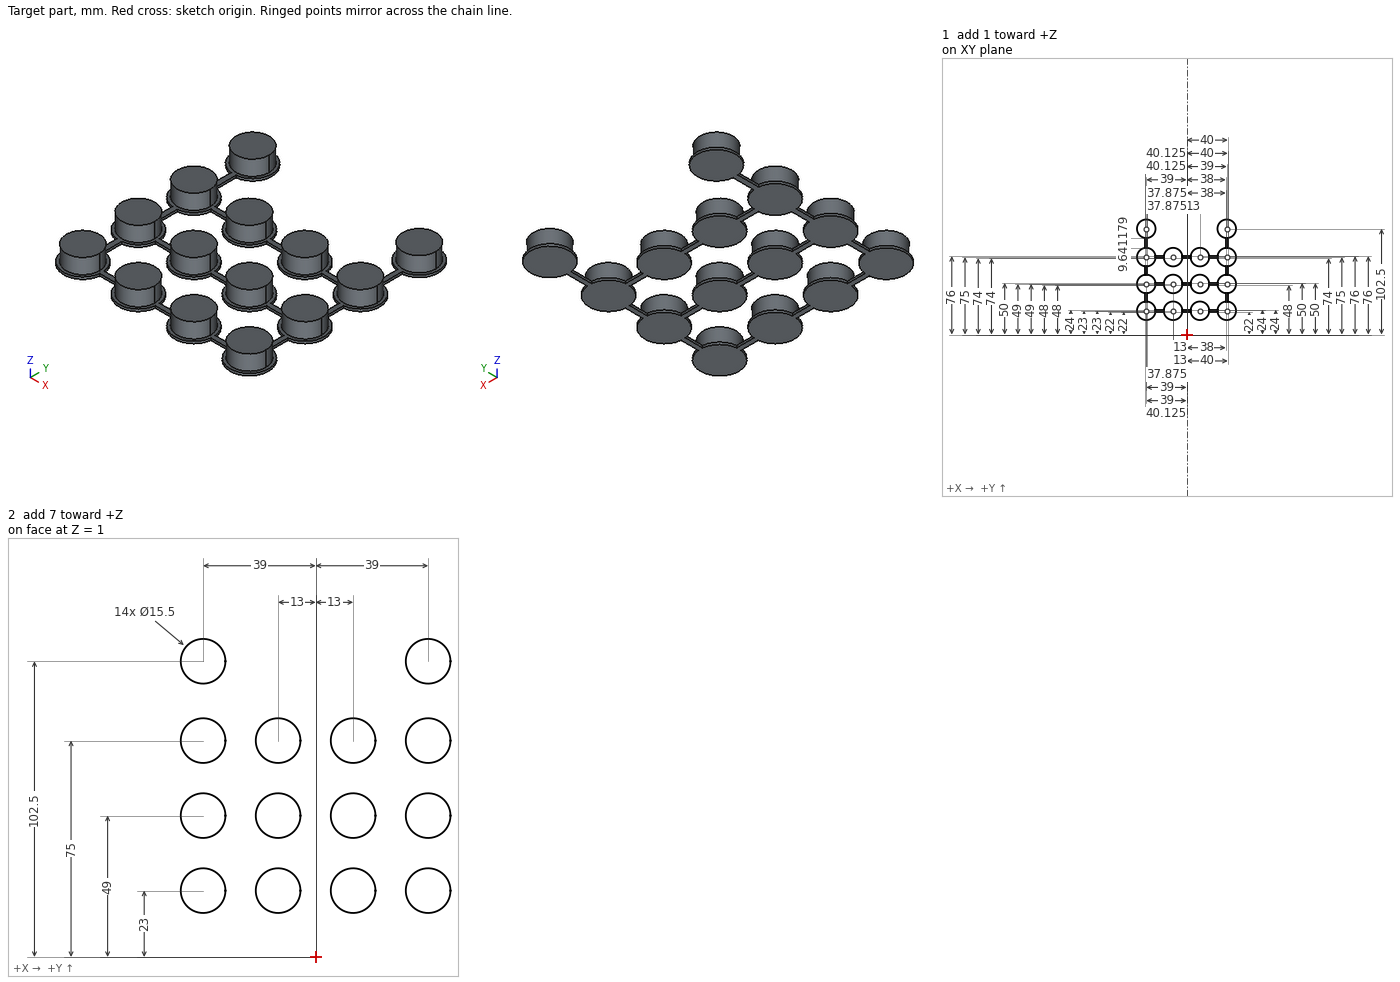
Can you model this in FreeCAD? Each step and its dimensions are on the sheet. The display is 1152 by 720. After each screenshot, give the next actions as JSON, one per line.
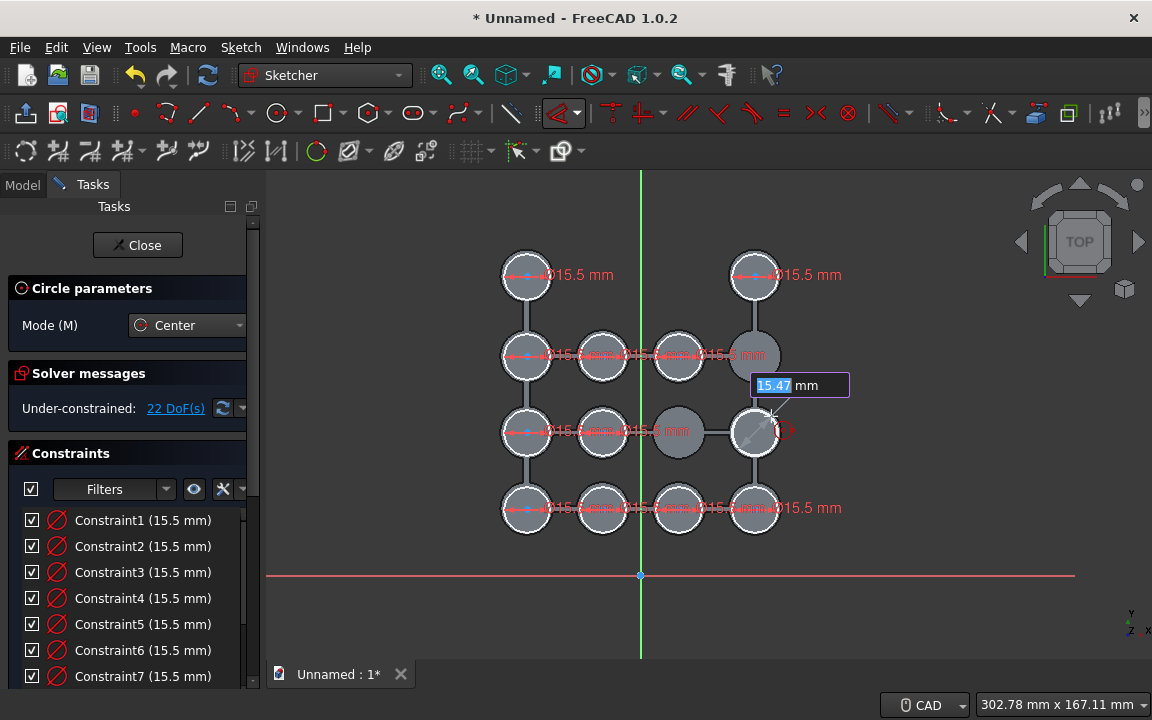
{"action": "type", "text": "15.5"}
{"action": "key", "text": "Return"}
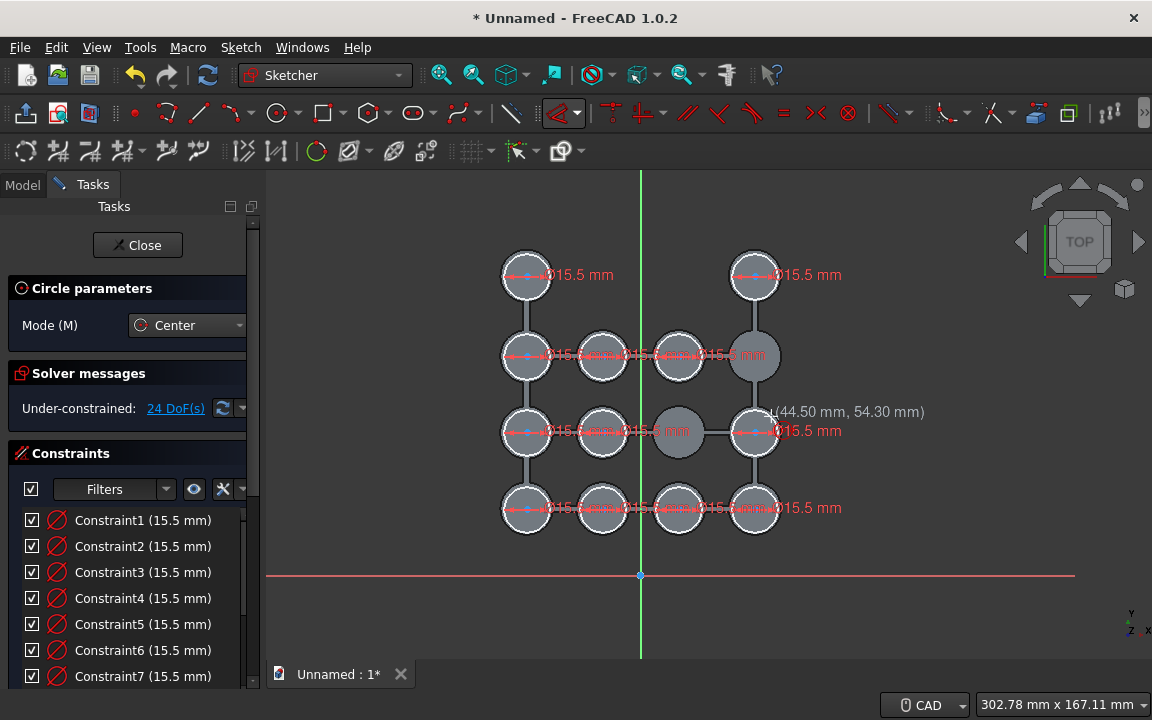
{"action": "left_click", "coordinate": [679, 432]}
{"action": "mouse_move", "coordinate": [695, 416]}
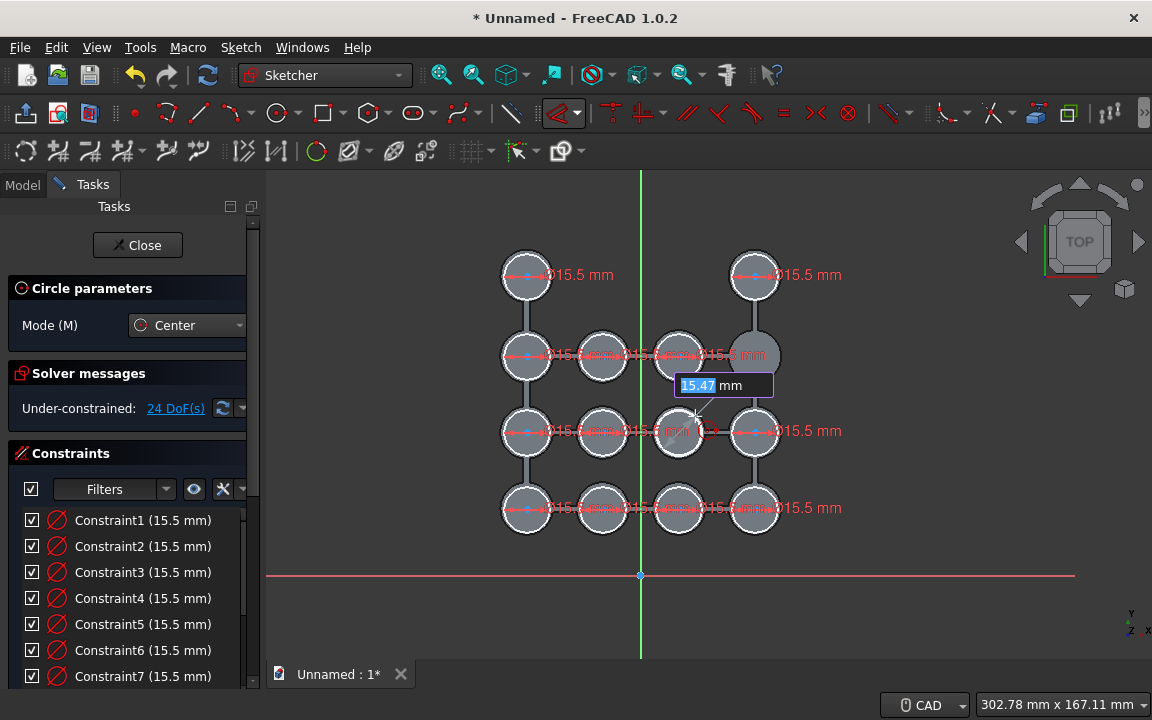
{"action": "type", "text": "15.5"}
{"action": "key", "text": "Return"}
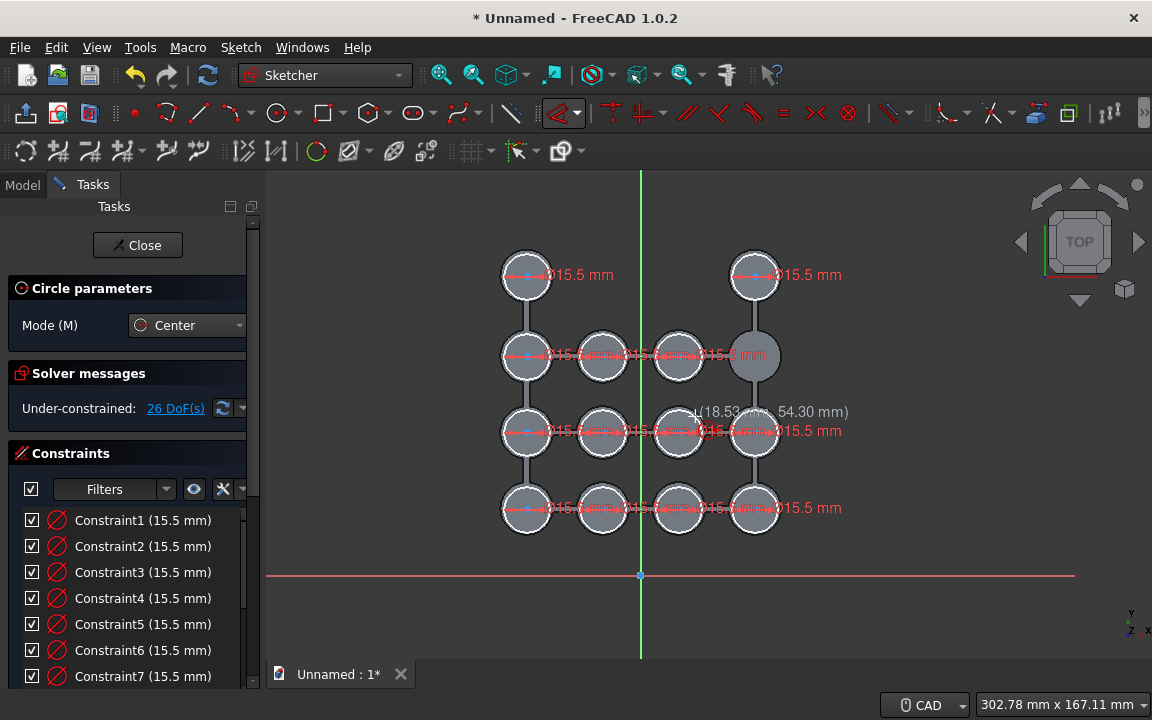
{"action": "left_click", "coordinate": [755, 356]}
{"action": "mouse_move", "coordinate": [771, 340]}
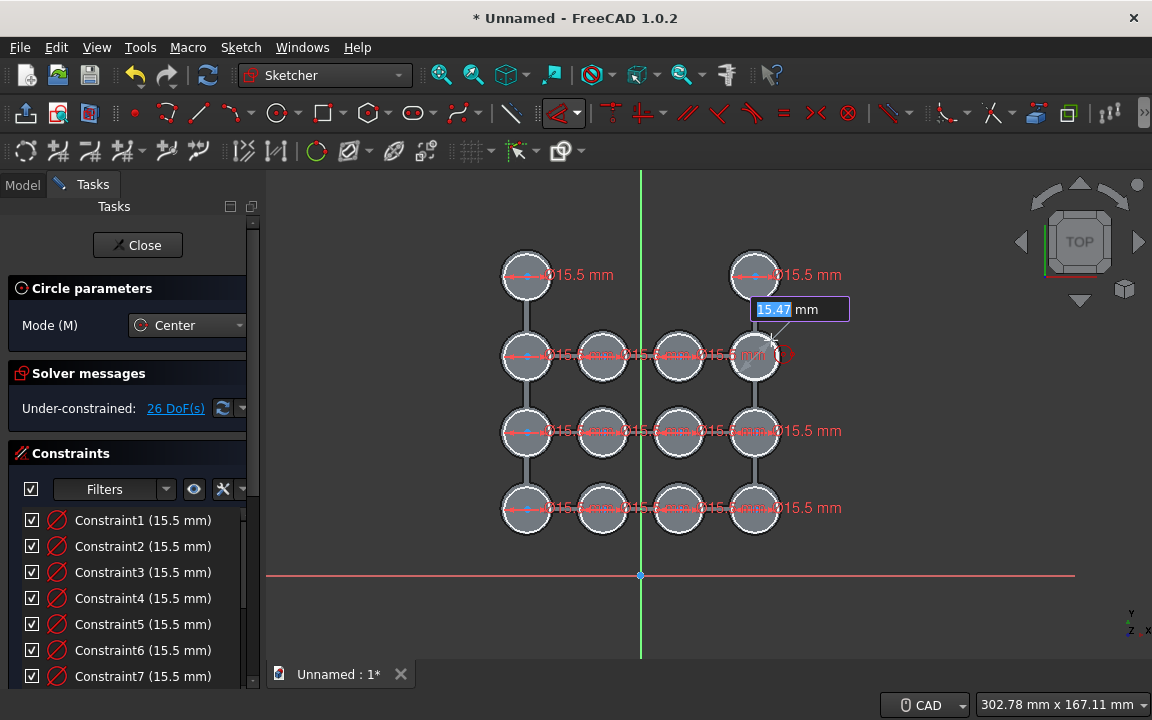
{"action": "type", "text": "15.5"}
{"action": "key", "text": "Return"}
{"action": "key", "text": "Escape"}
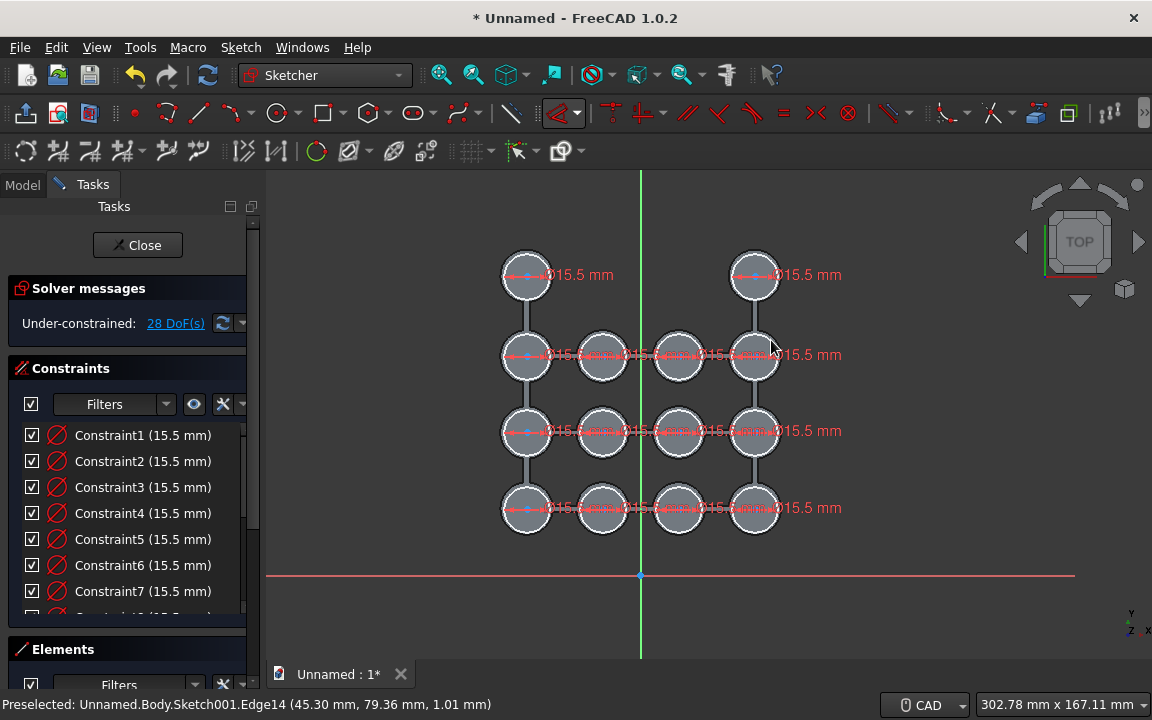
{"action": "left_click", "coordinate": [527, 277]}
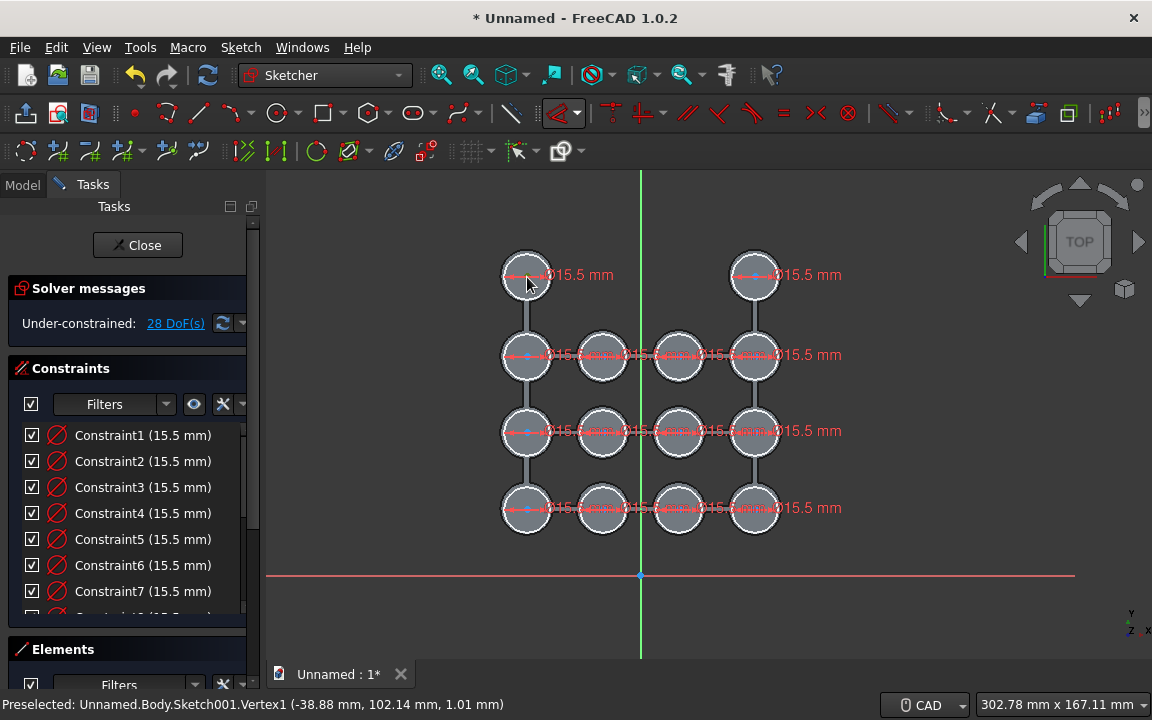
{"action": "left_click", "coordinate": [527, 357]}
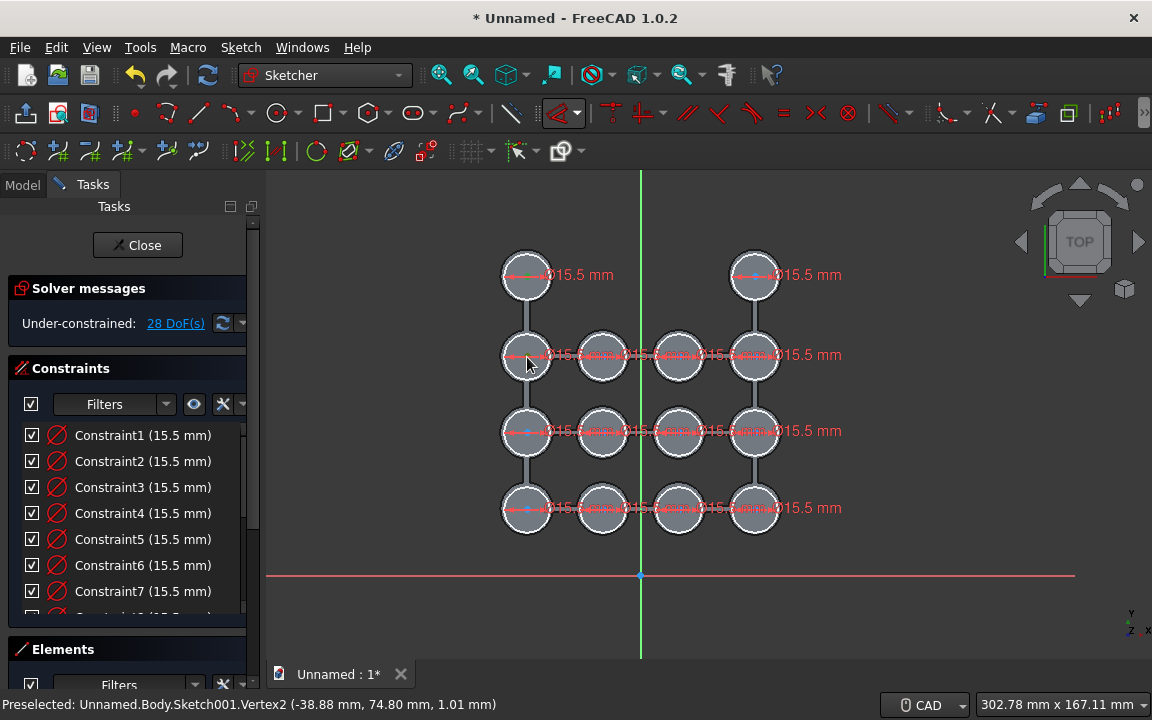
{"action": "left_click", "coordinate": [666, 114]}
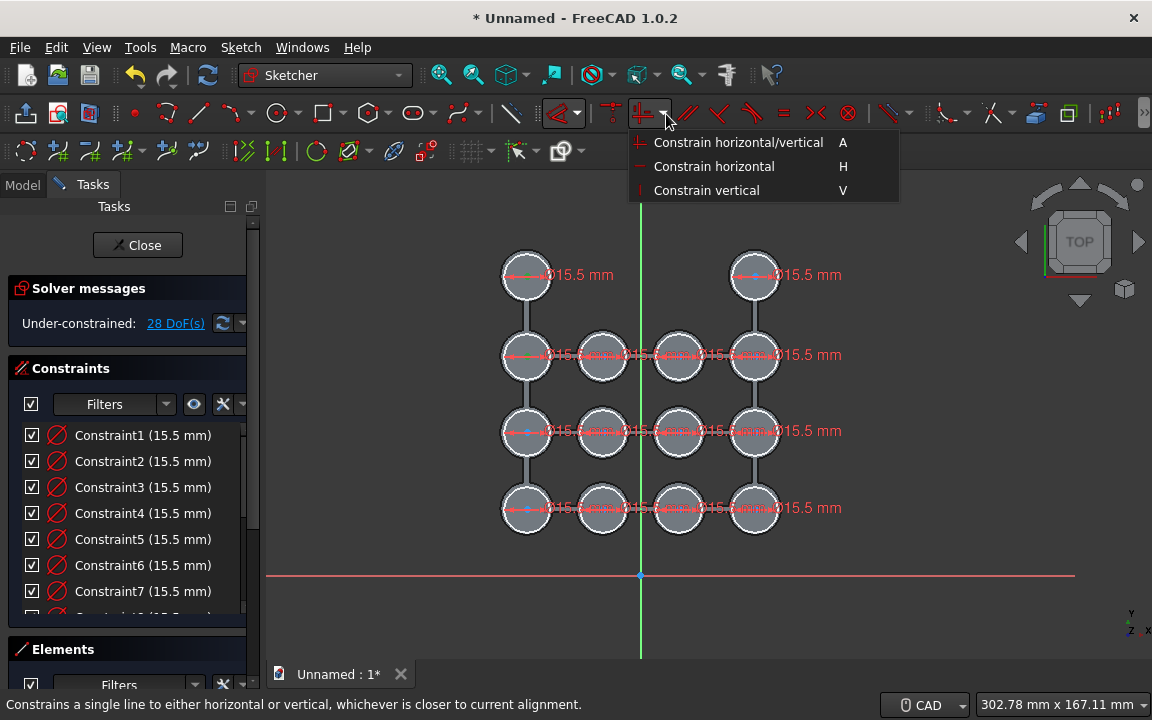
{"action": "left_click", "coordinate": [764, 190]}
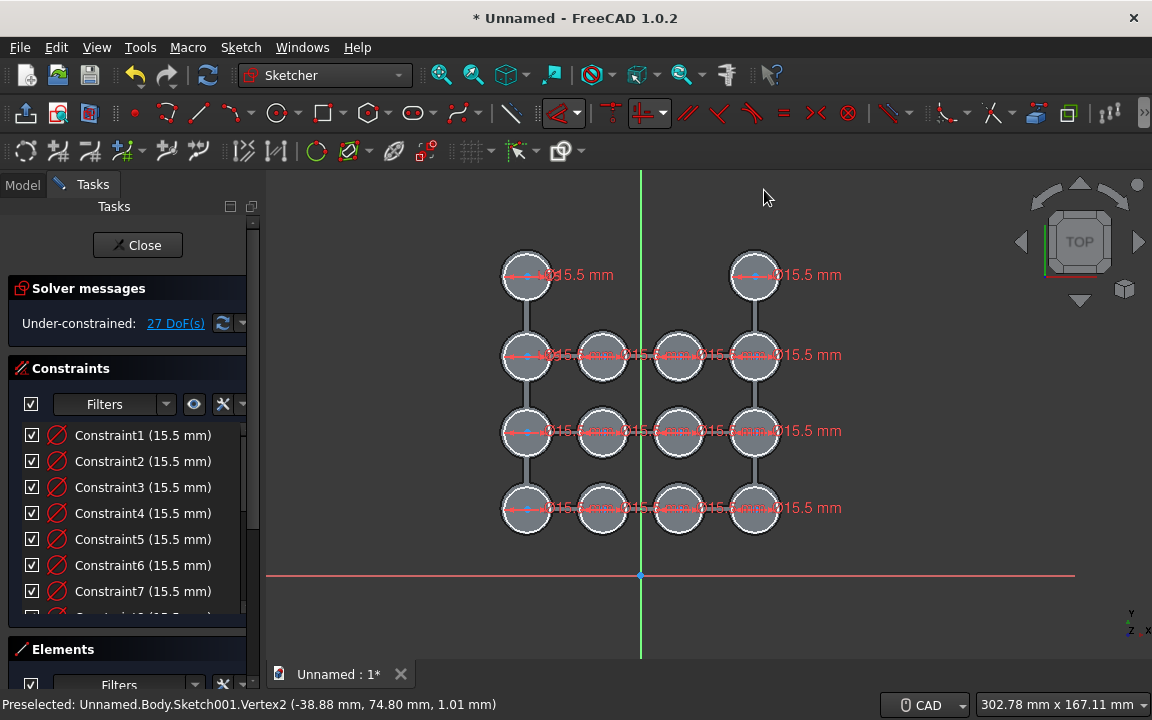
{"action": "left_click", "coordinate": [527, 357]}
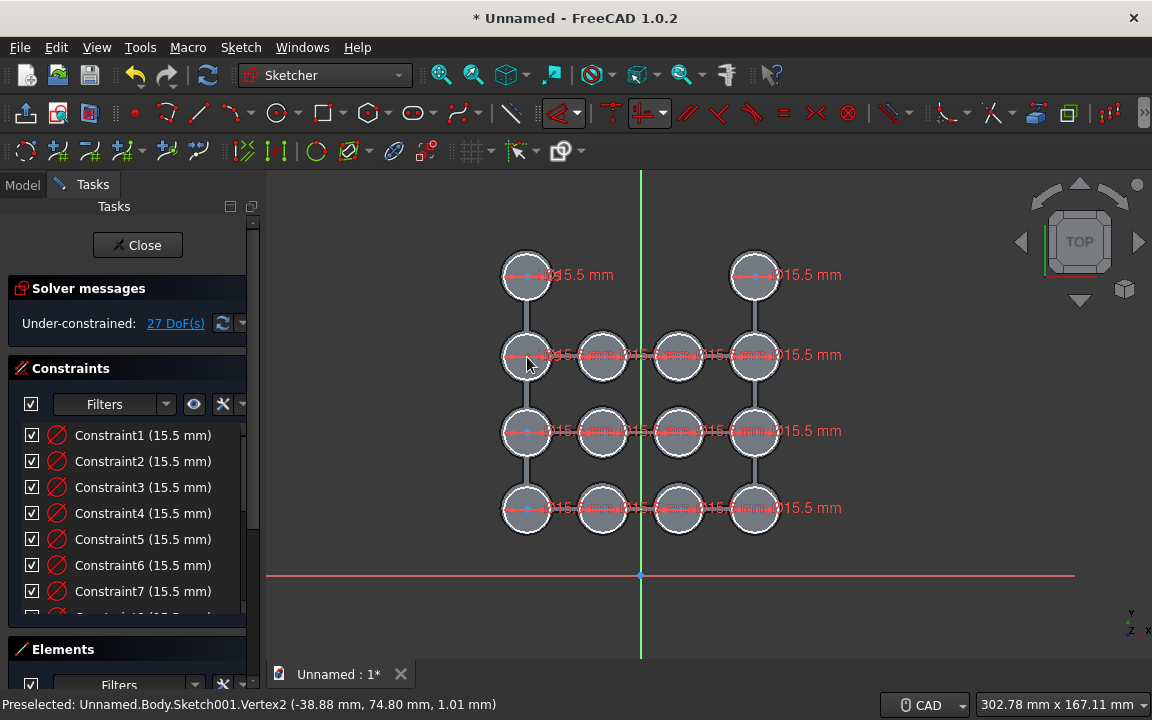
{"action": "left_click", "coordinate": [527, 433]}